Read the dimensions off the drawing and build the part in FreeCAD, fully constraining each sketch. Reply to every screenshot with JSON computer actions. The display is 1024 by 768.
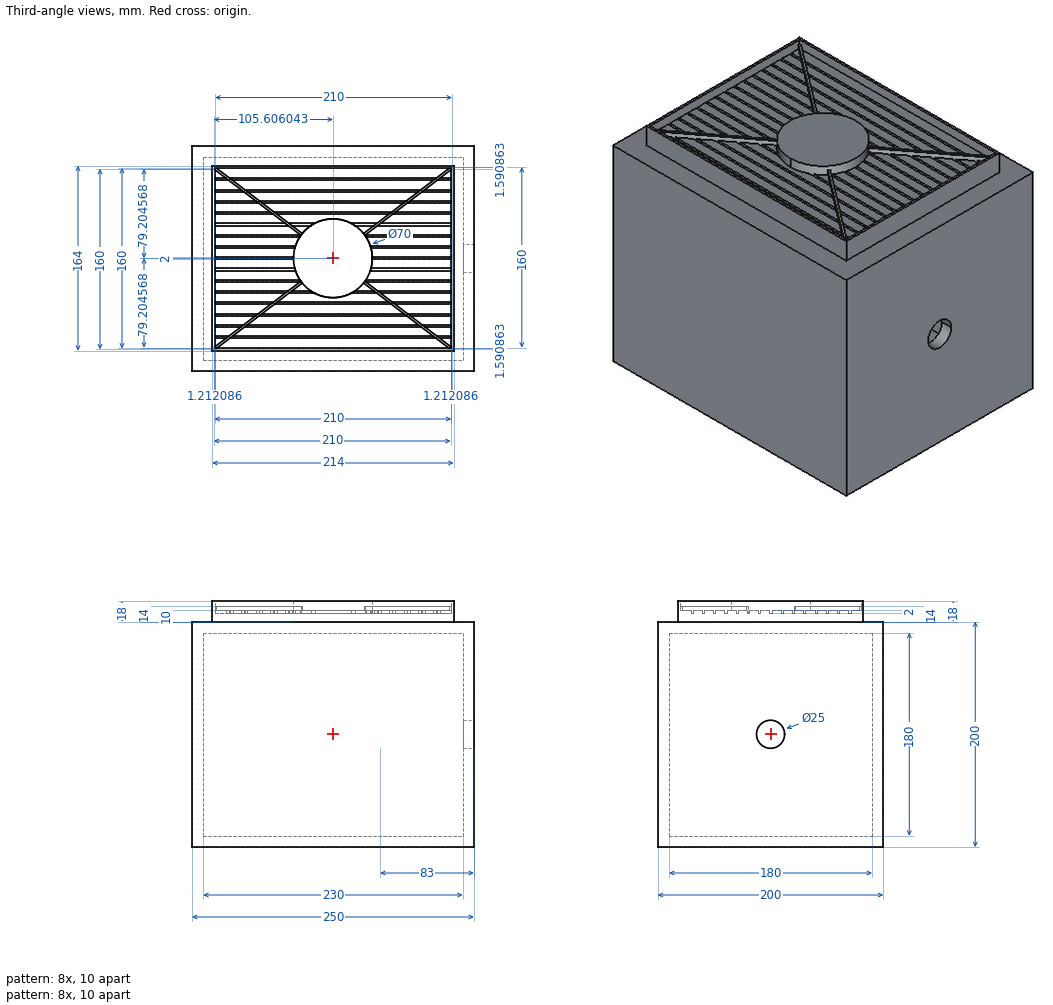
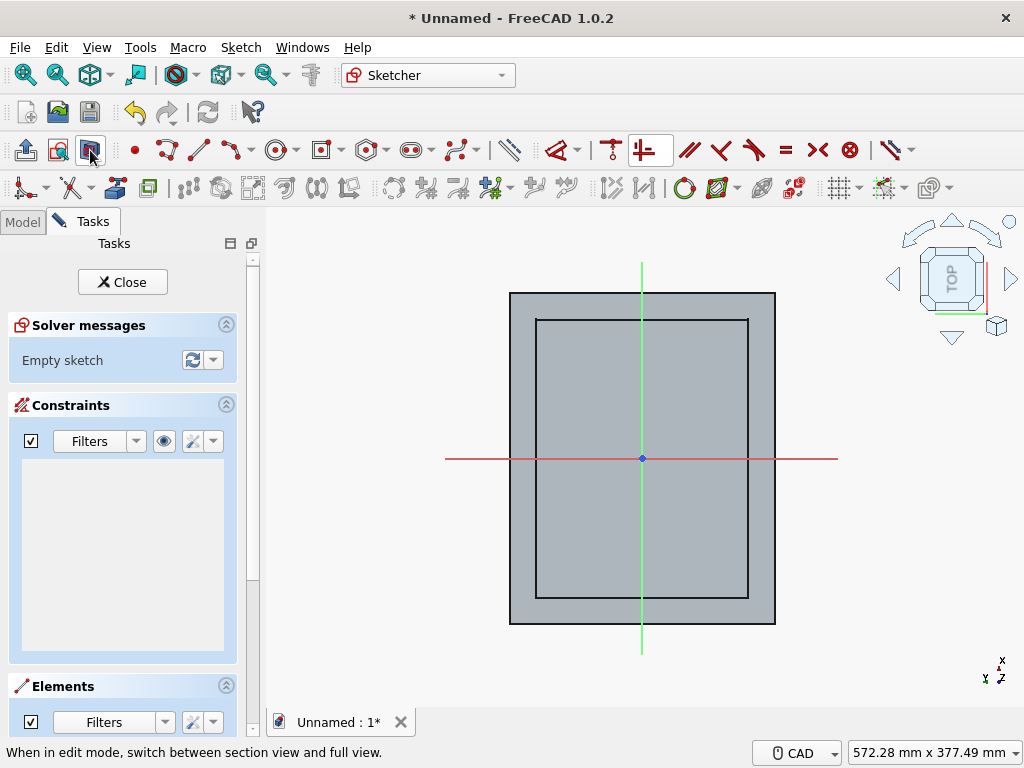
{"action": "scroll", "coordinate": [671, 459], "scroll_direction": "up", "scroll_amount": 6}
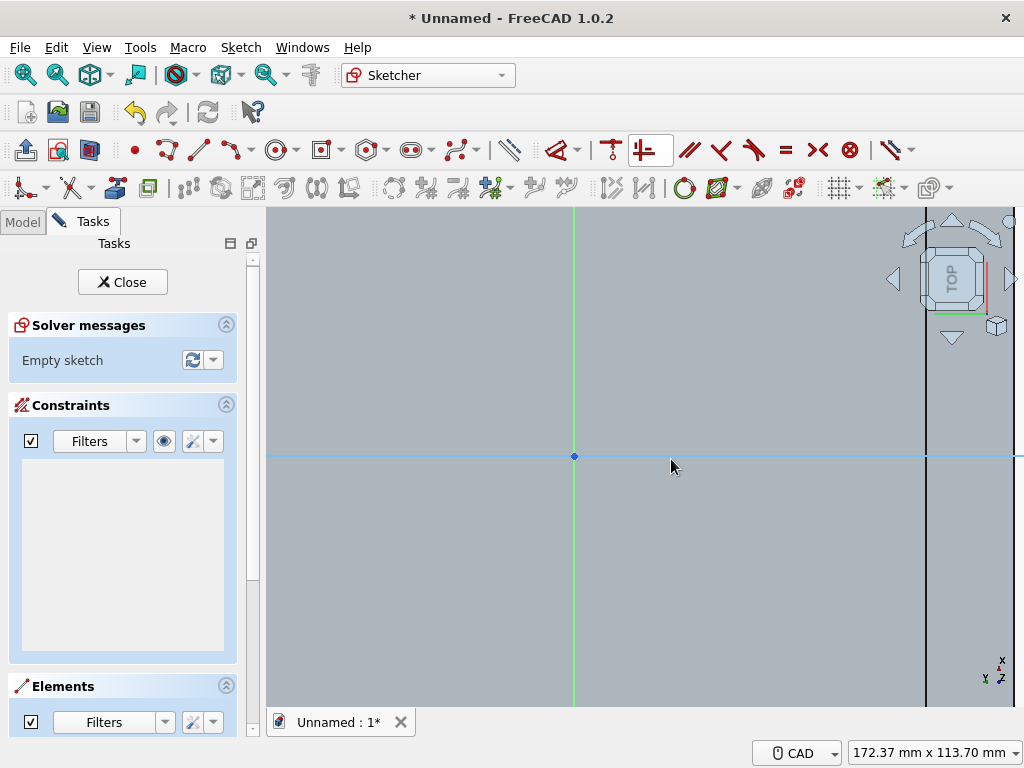
{"action": "left_click", "coordinate": [276, 150]}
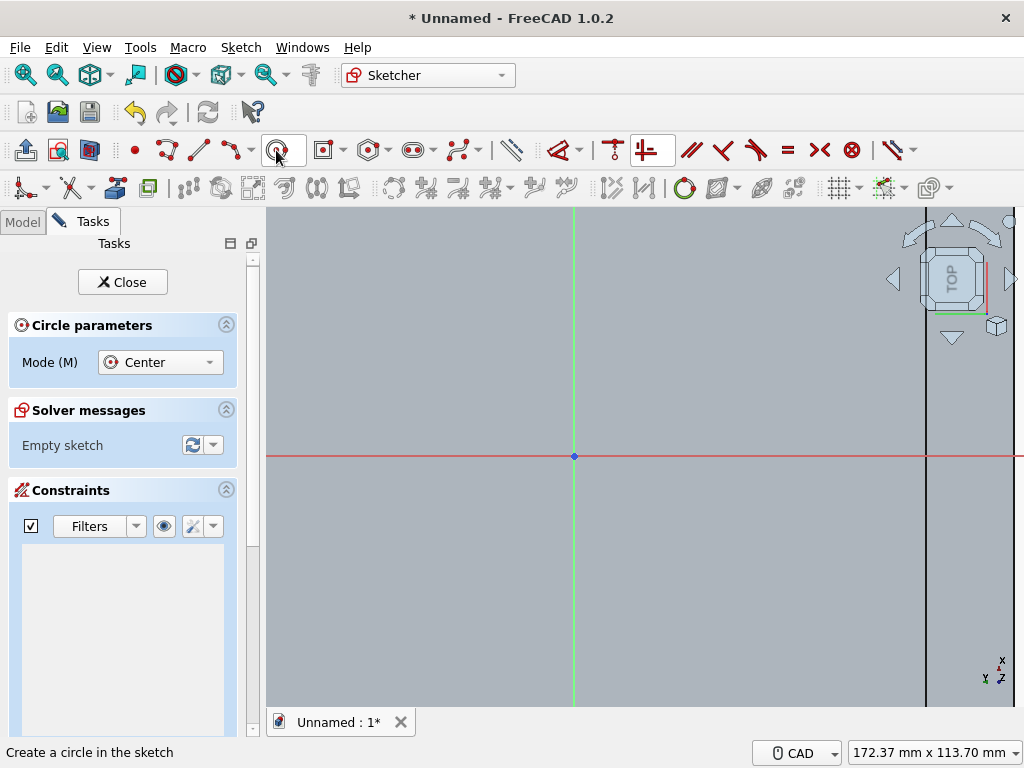
{"action": "left_click", "coordinate": [574, 456]}
{"action": "left_click", "coordinate": [683, 348]}
{"action": "key", "text": "Escape"}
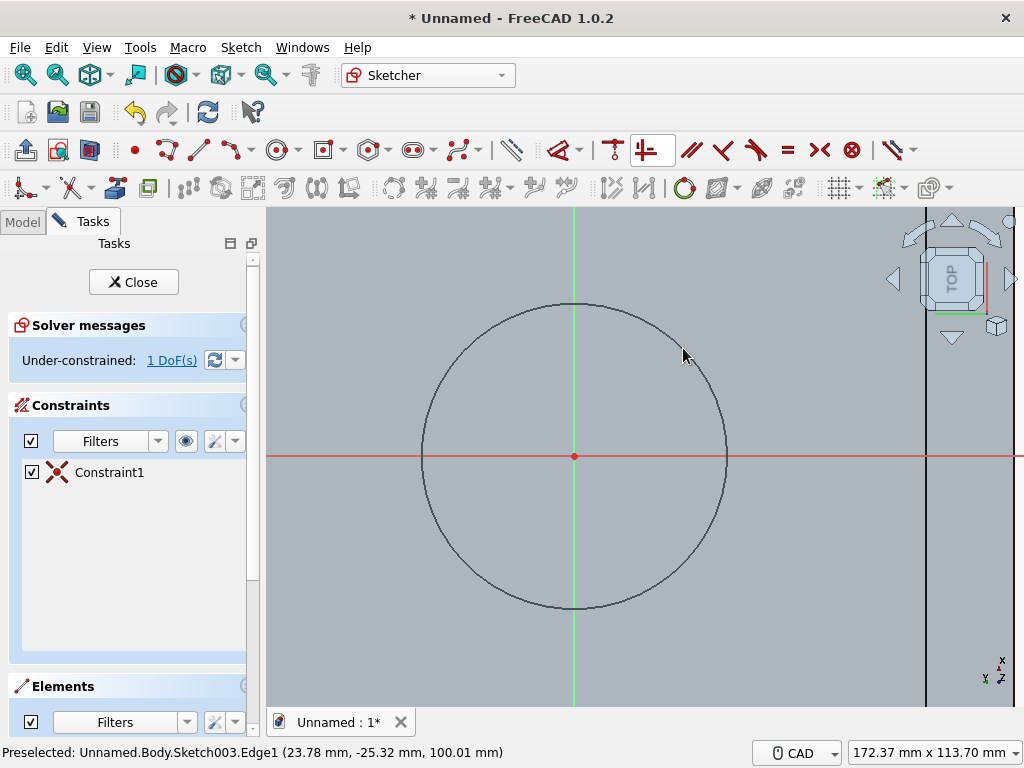
{"action": "left_click", "coordinate": [558, 150]}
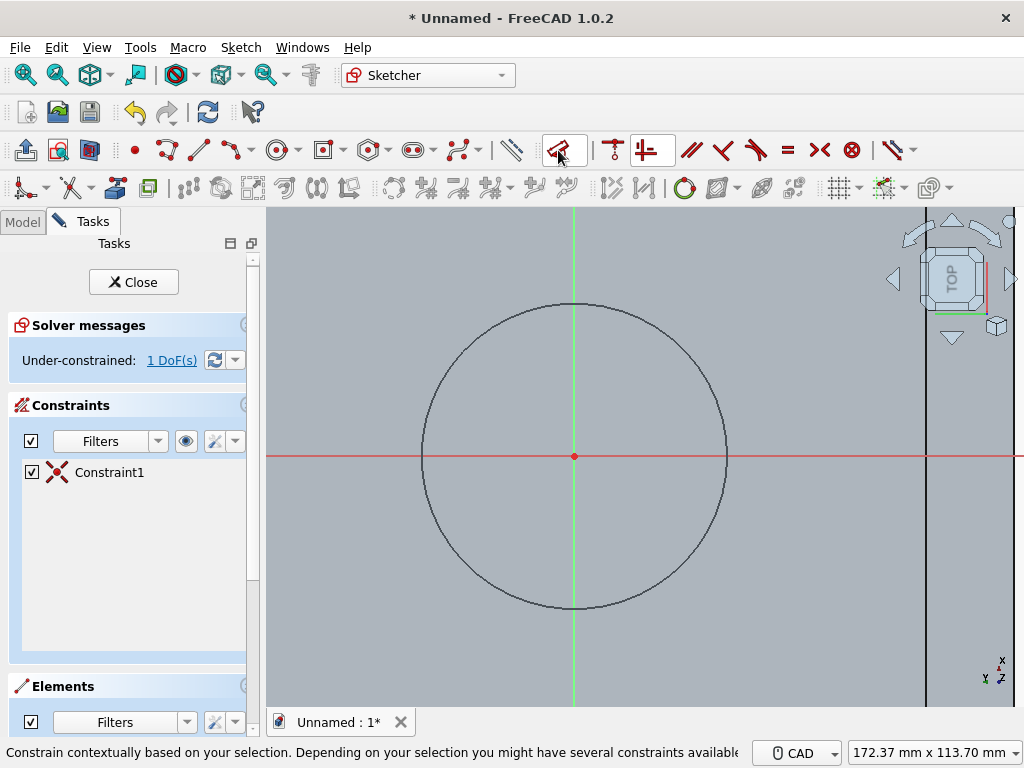
{"action": "left_click", "coordinate": [682, 348]}
{"action": "left_click", "coordinate": [705, 325]}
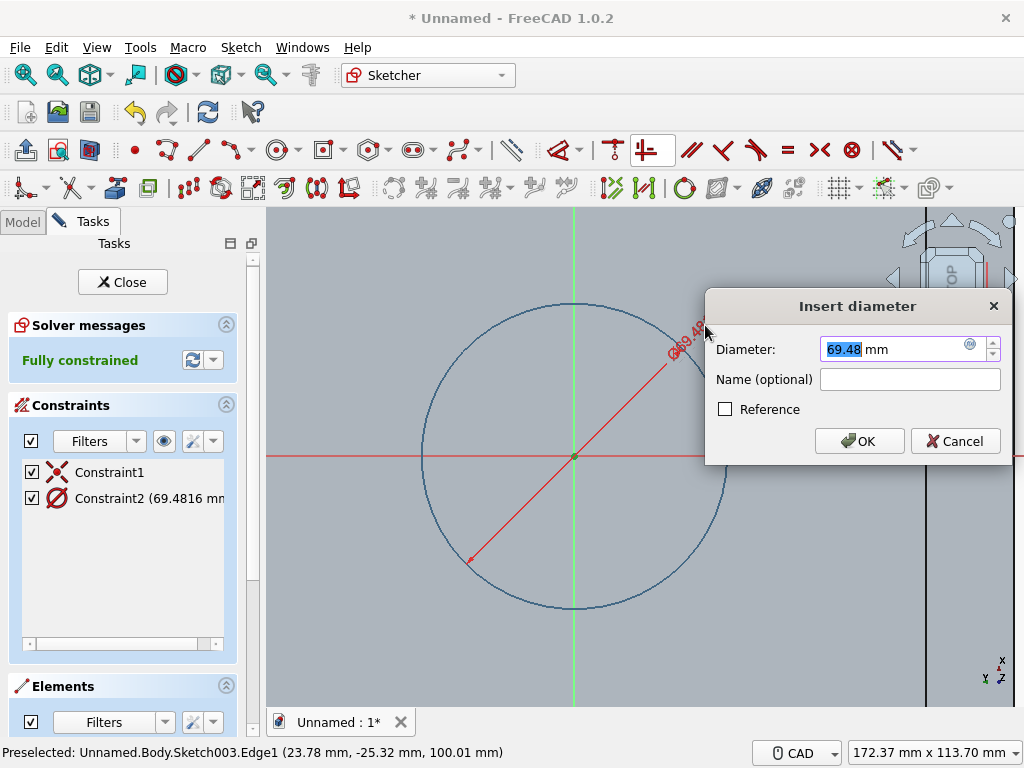
{"action": "type", "text": "70"}
{"action": "key", "text": "Return"}
{"action": "key", "text": "Escape"}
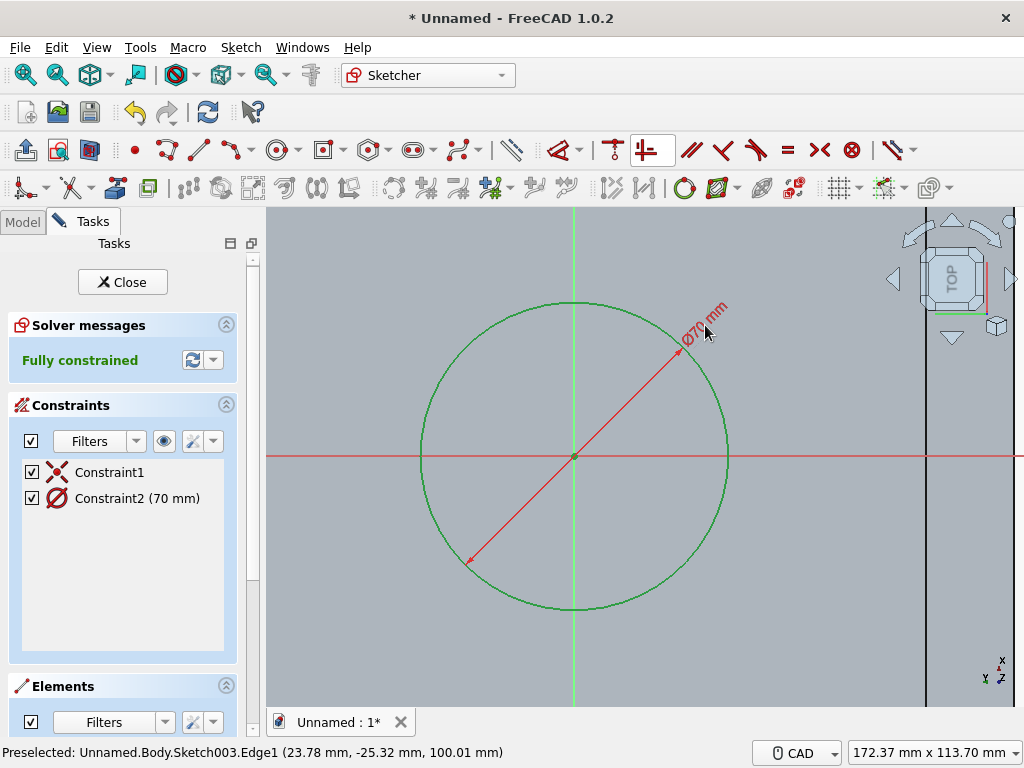
{"action": "left_click", "coordinate": [123, 282]}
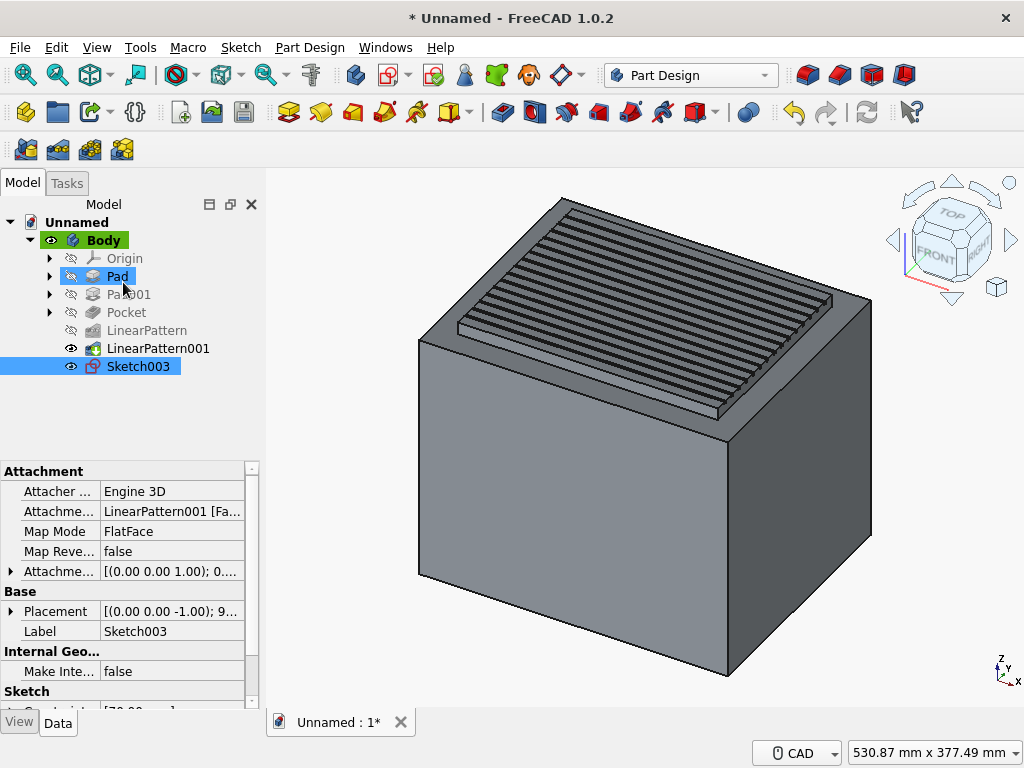
{"action": "left_click", "coordinate": [290, 112]}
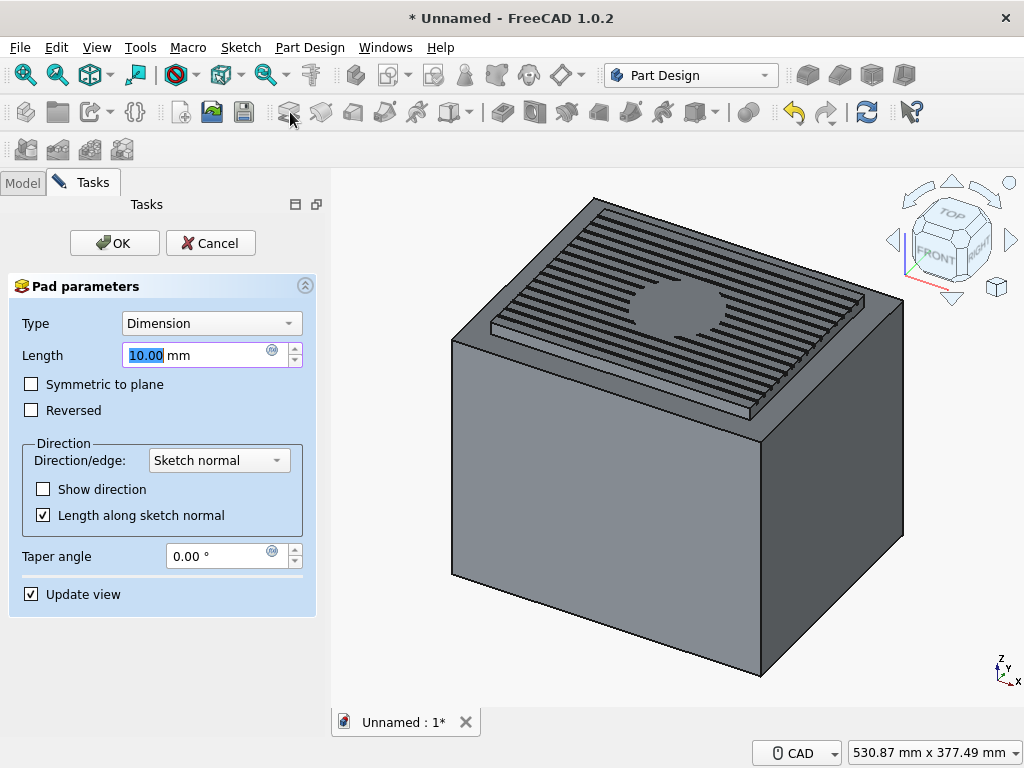
{"action": "type", "text": "18"}
{"action": "key", "text": "Tab"}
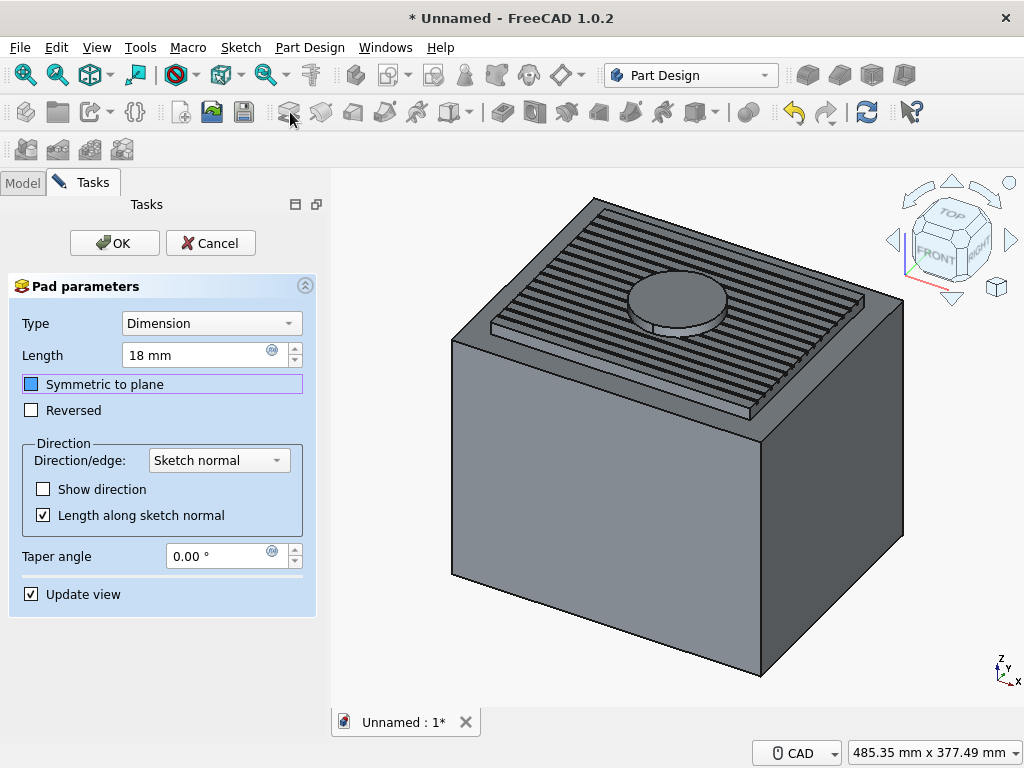
{"action": "left_click", "coordinate": [115, 243]}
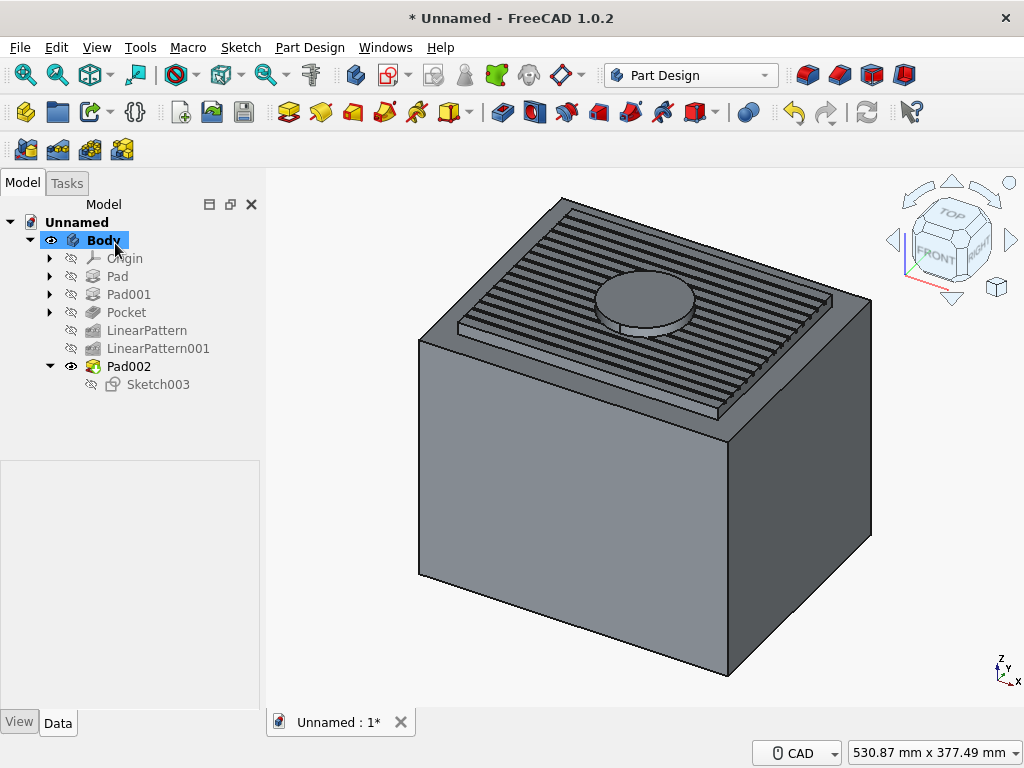
{"action": "left_click", "coordinate": [716, 424]}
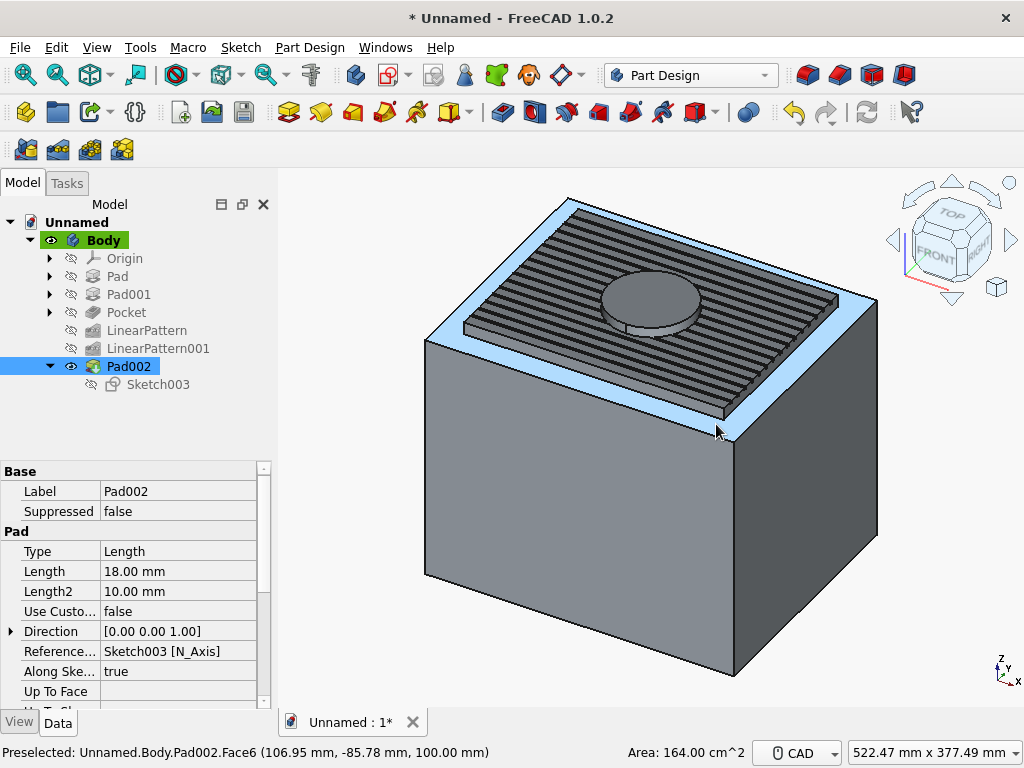
{"action": "left_click", "coordinate": [388, 76]}